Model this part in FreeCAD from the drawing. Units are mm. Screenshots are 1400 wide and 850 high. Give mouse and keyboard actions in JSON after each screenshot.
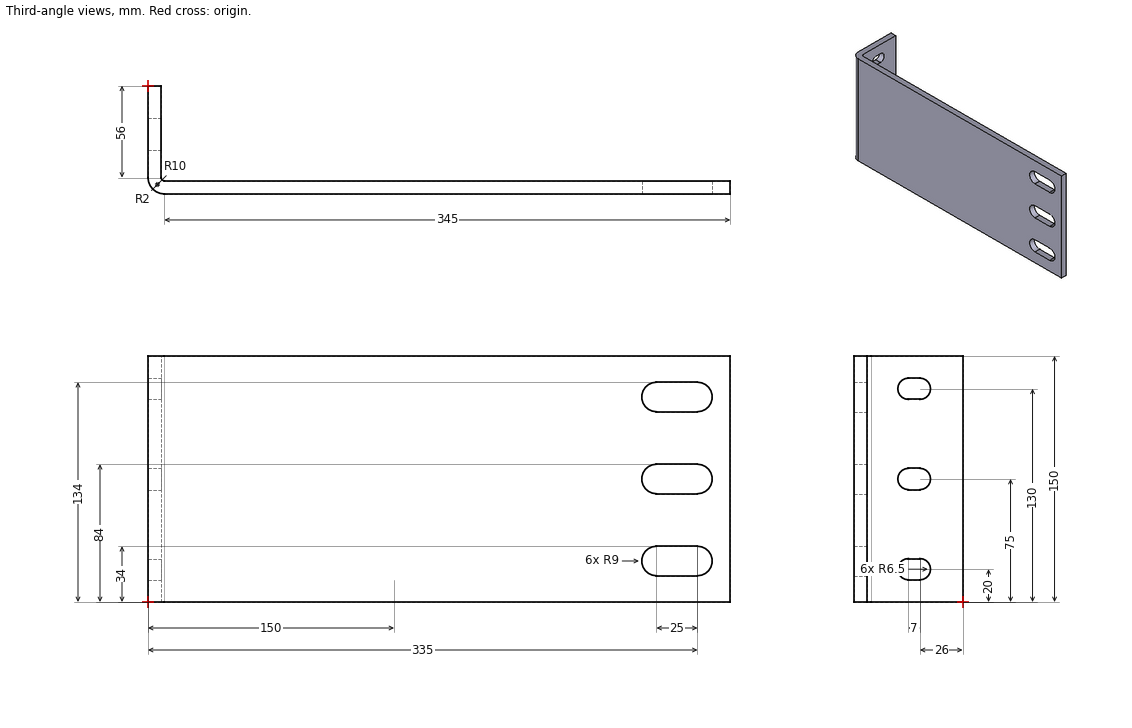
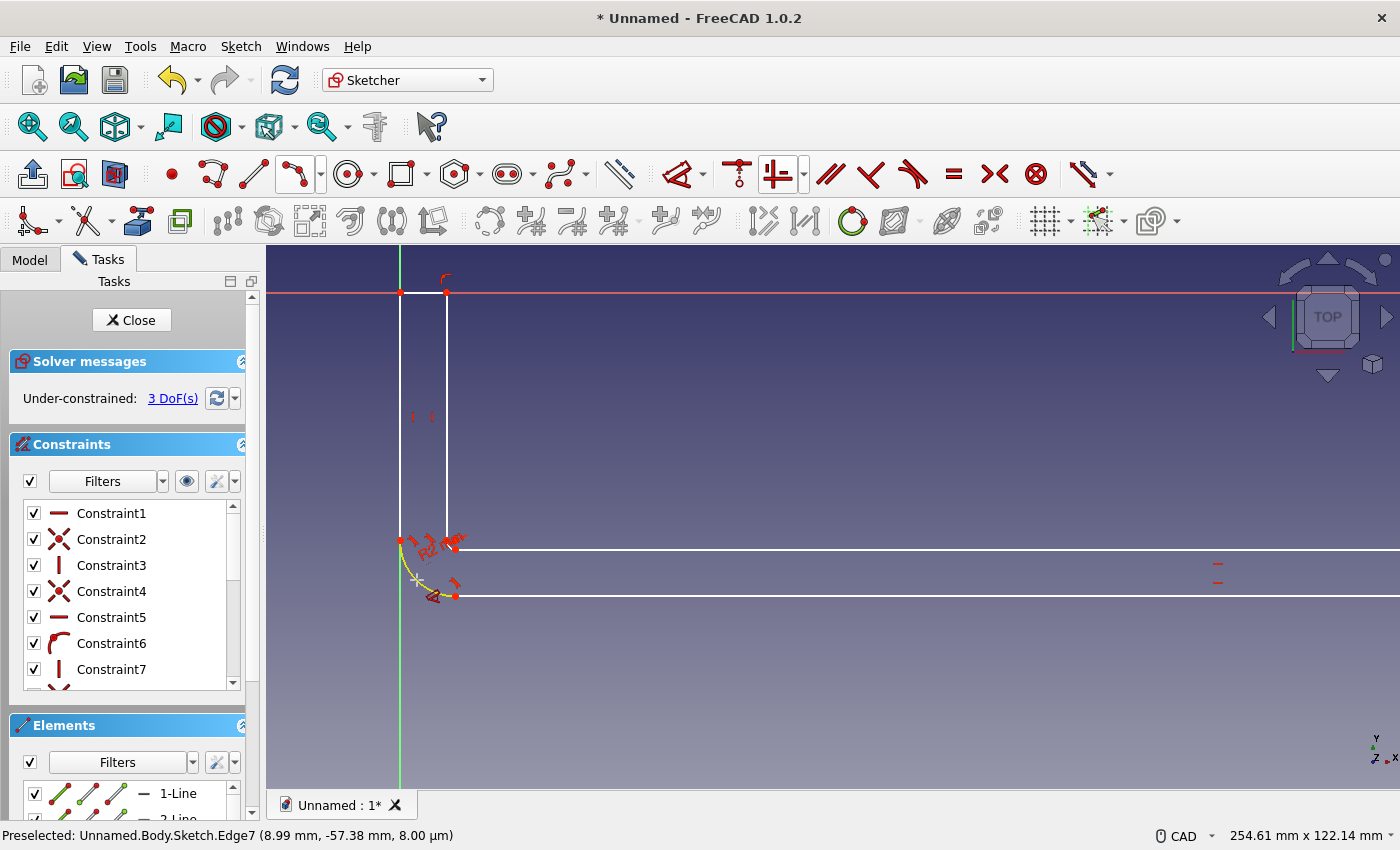
{"action": "left_click", "coordinate": [416, 580]}
{"action": "left_click", "coordinate": [430, 625]}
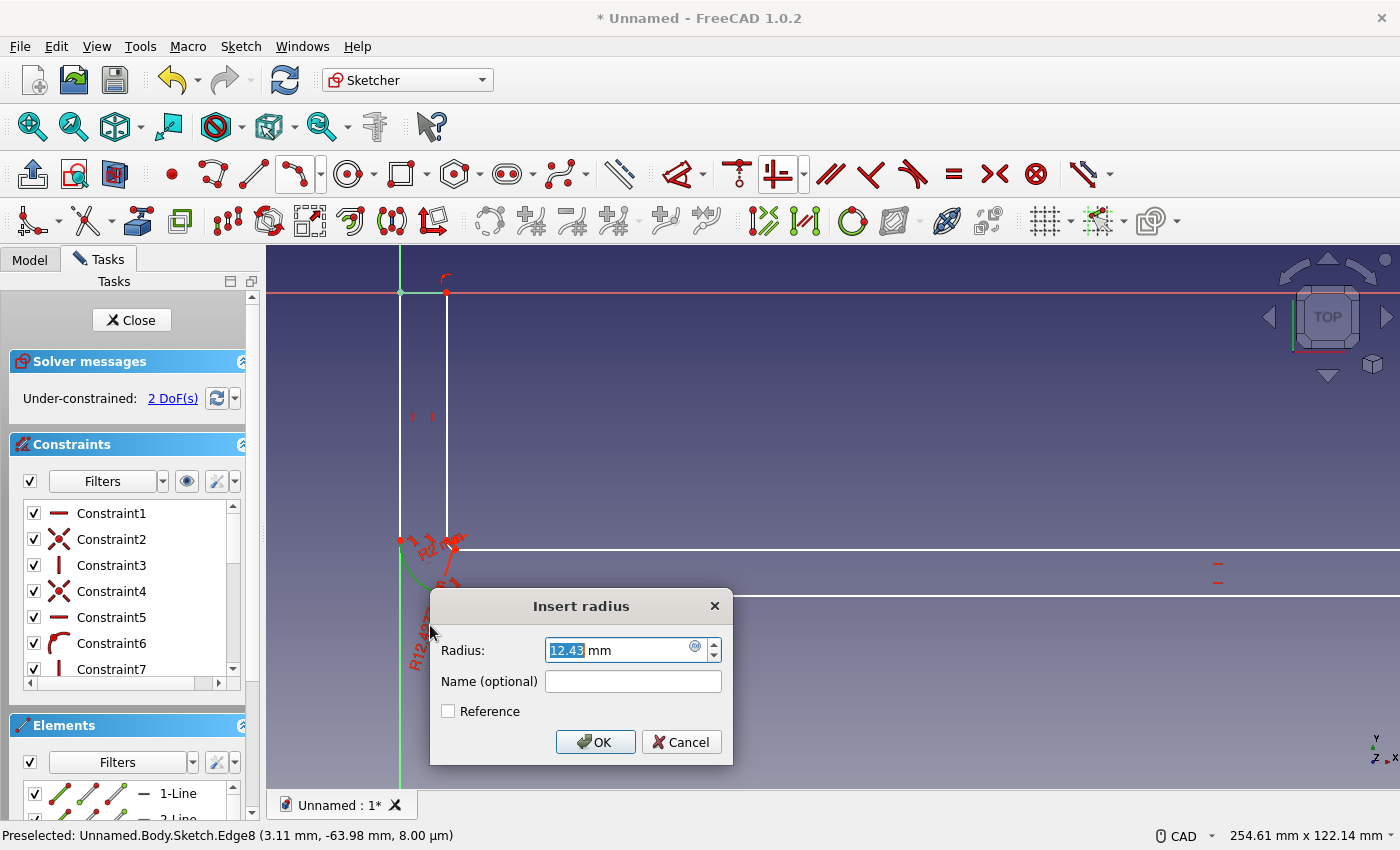
{"action": "type", "text": "10"}
{"action": "key", "text": "Return"}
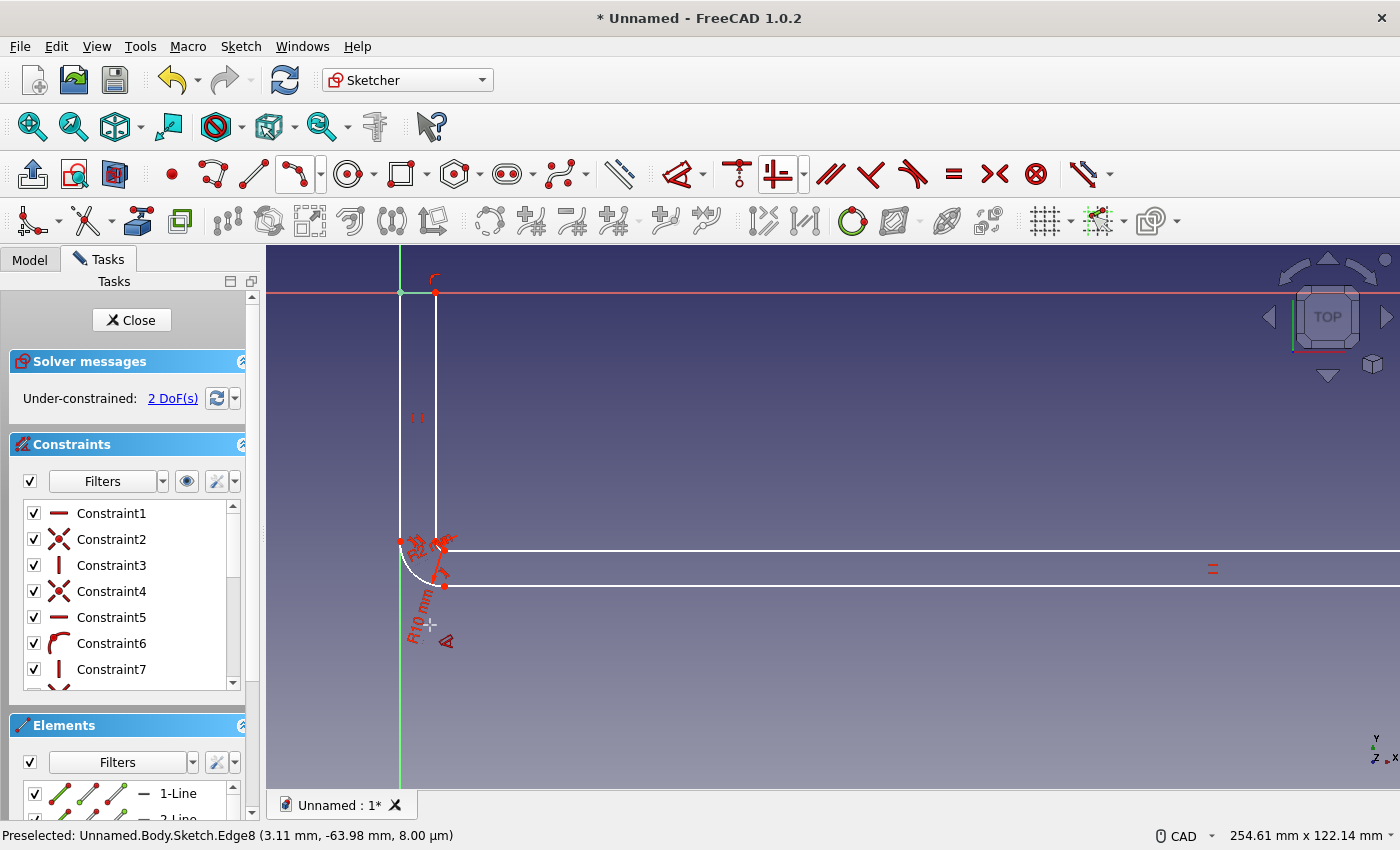
{"action": "left_click", "coordinate": [436, 467]}
{"action": "left_click", "coordinate": [470, 417]}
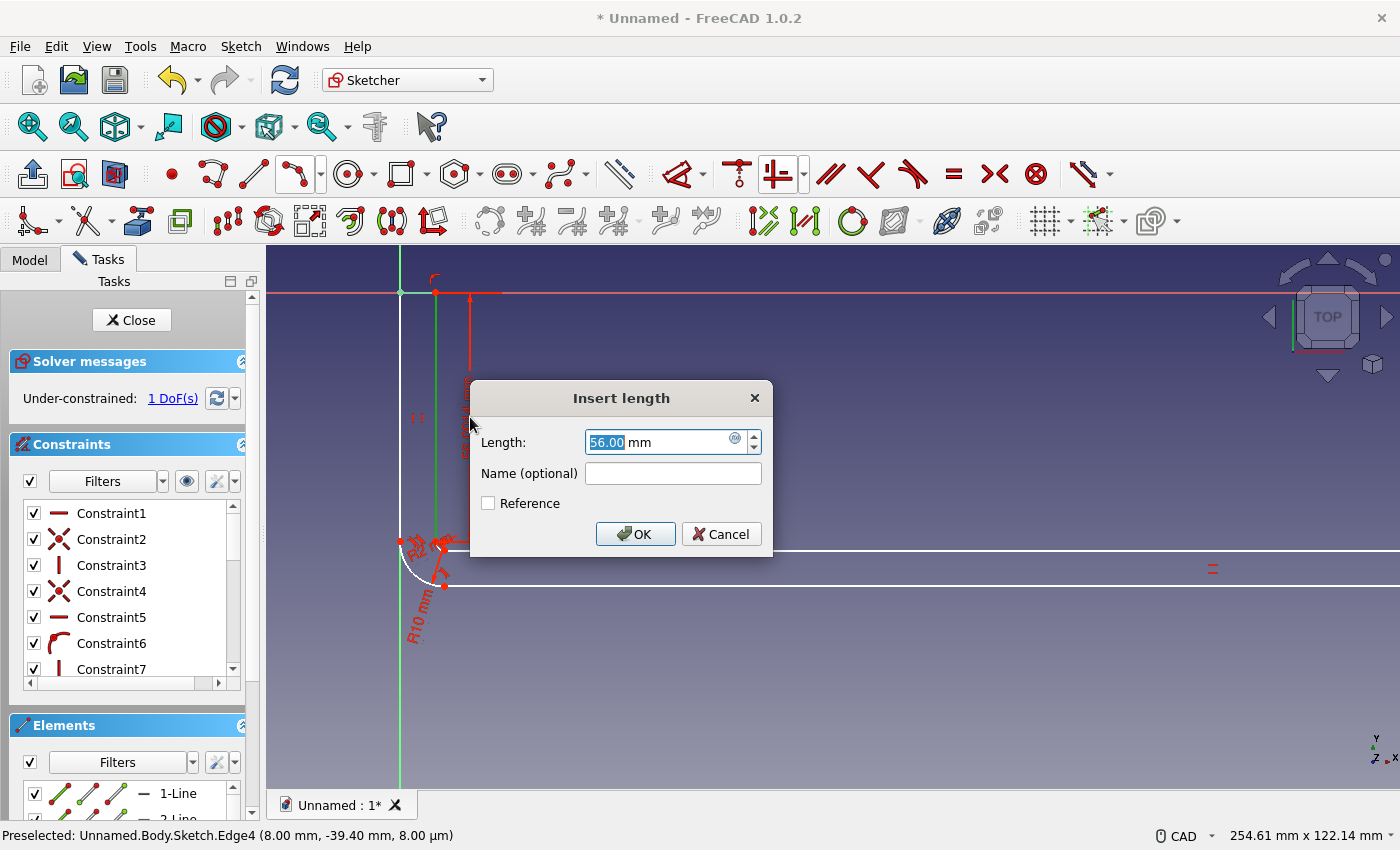
{"action": "type", "text": "56"}
{"action": "key", "text": "Return"}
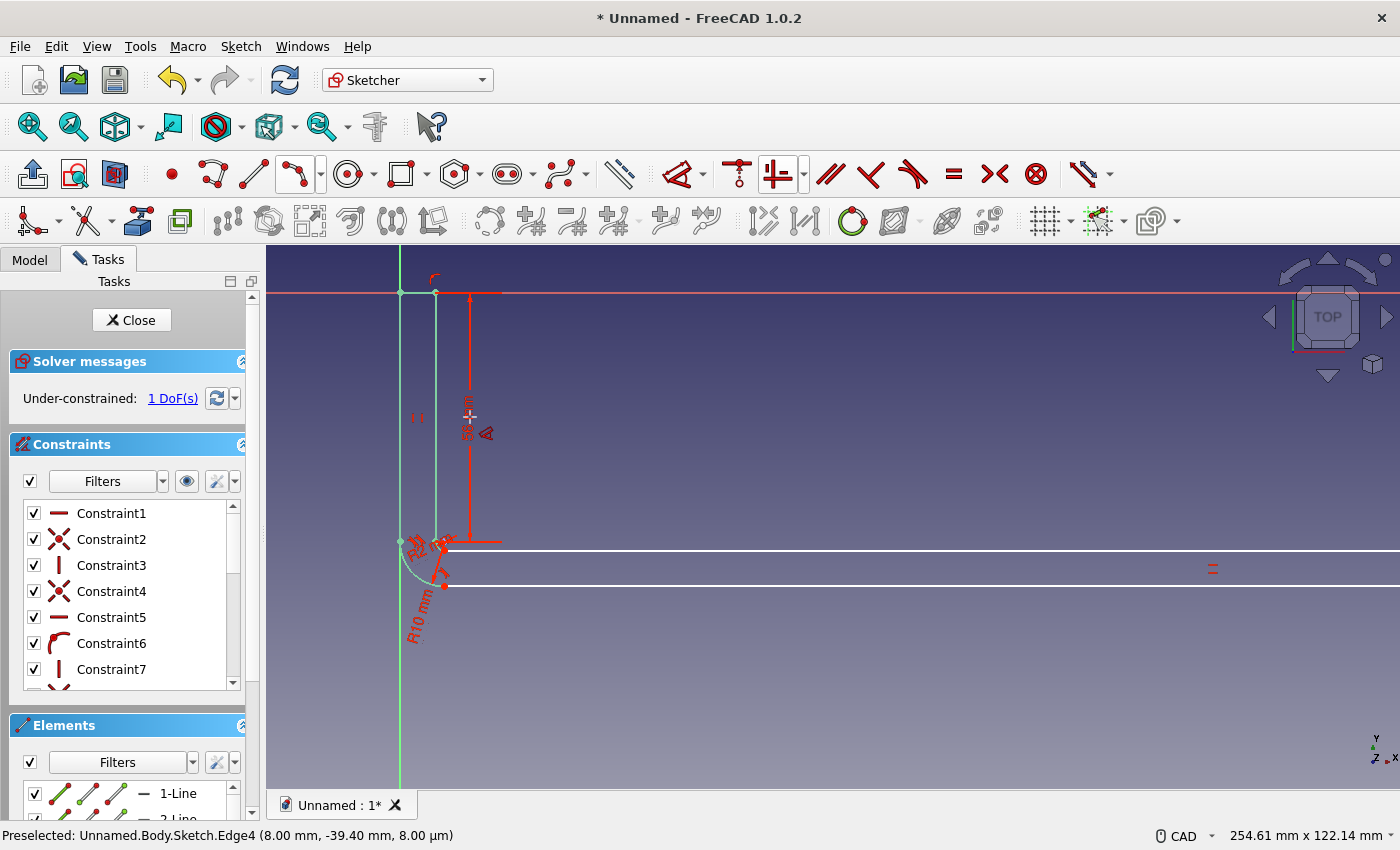
{"action": "left_click", "coordinate": [906, 586]}
{"action": "left_click", "coordinate": [840, 620]}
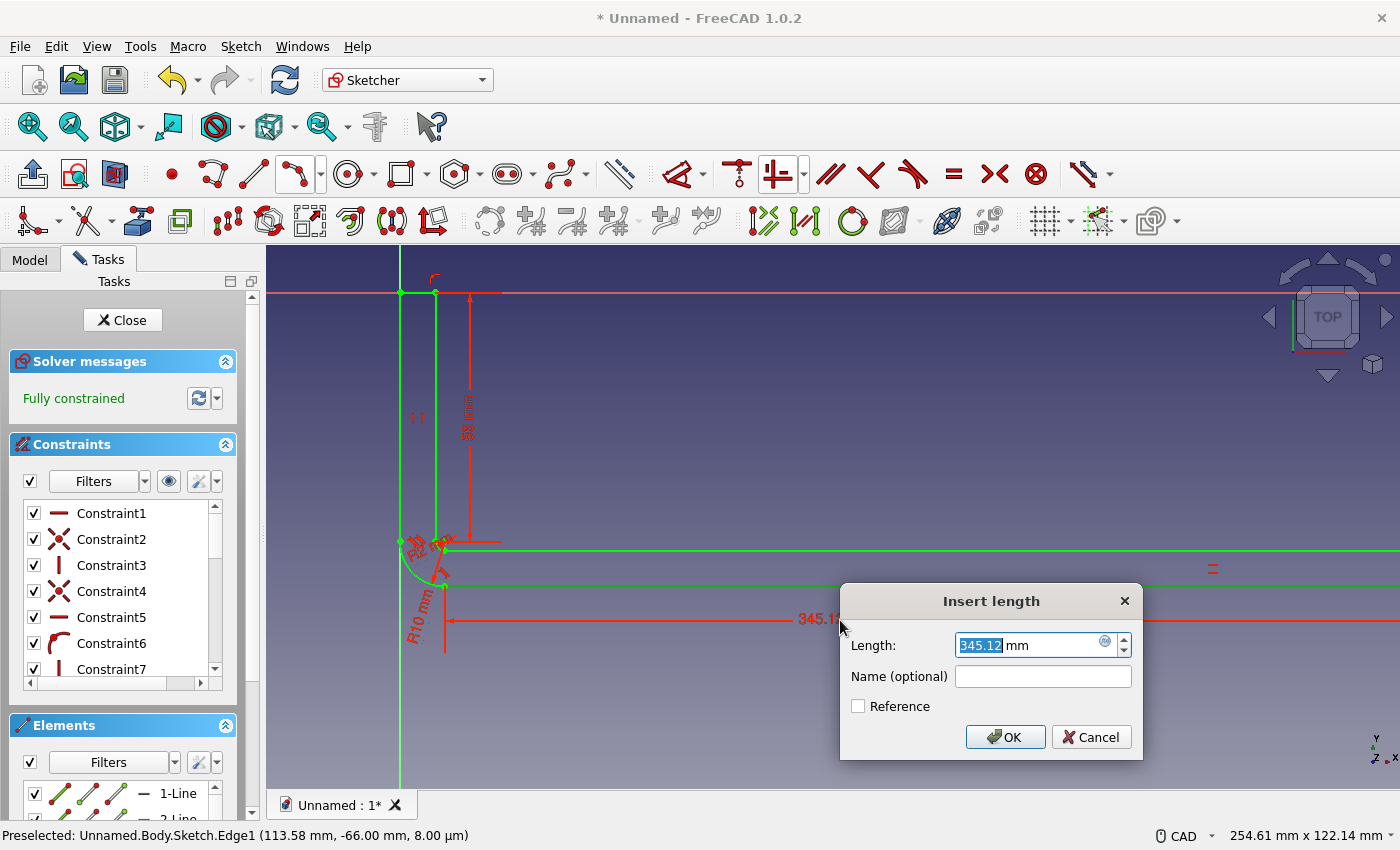
{"action": "type", "text": "345"}
{"action": "key", "text": "Return"}
{"action": "key", "text": "Escape"}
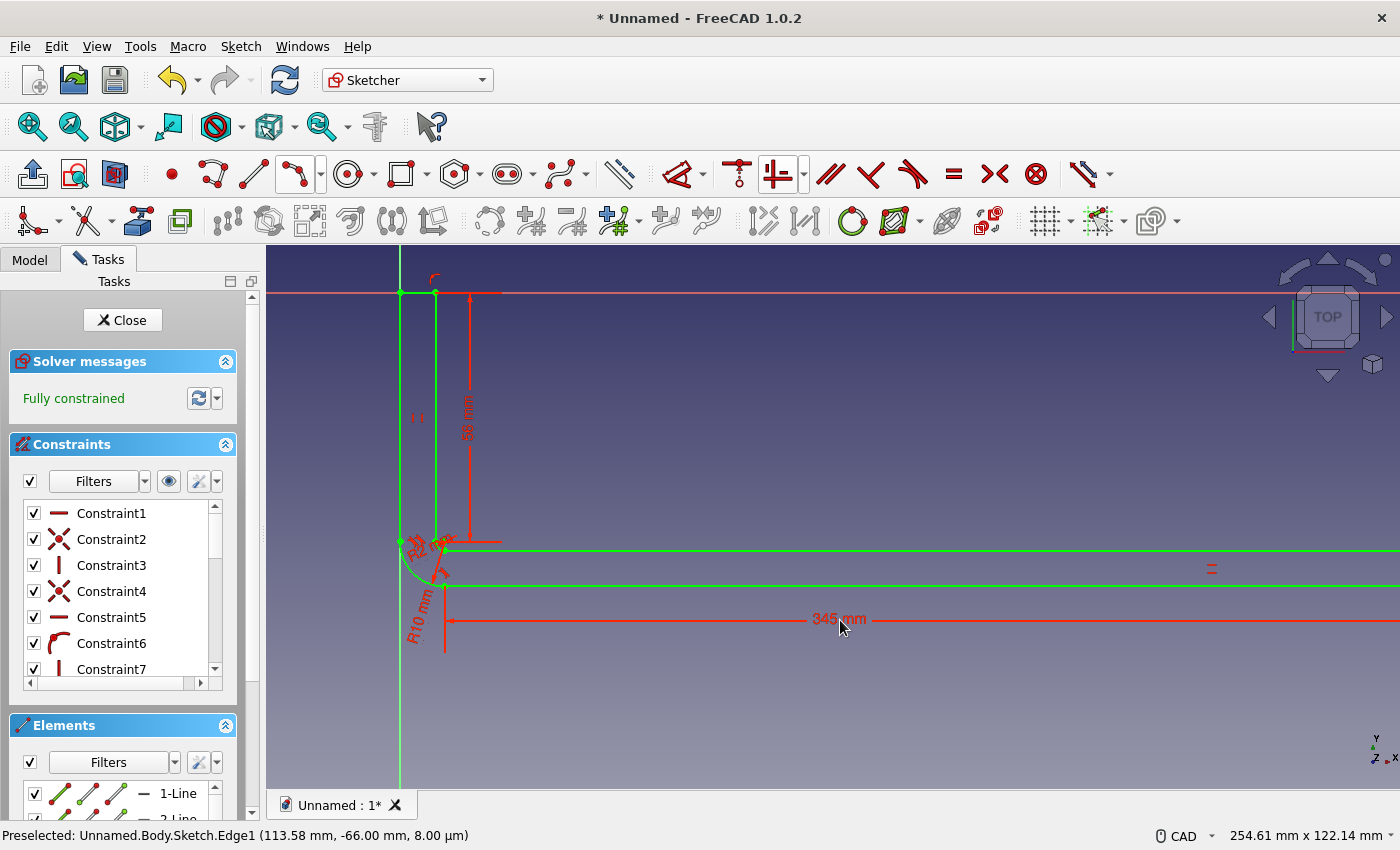
{"action": "left_click", "coordinate": [123, 320]}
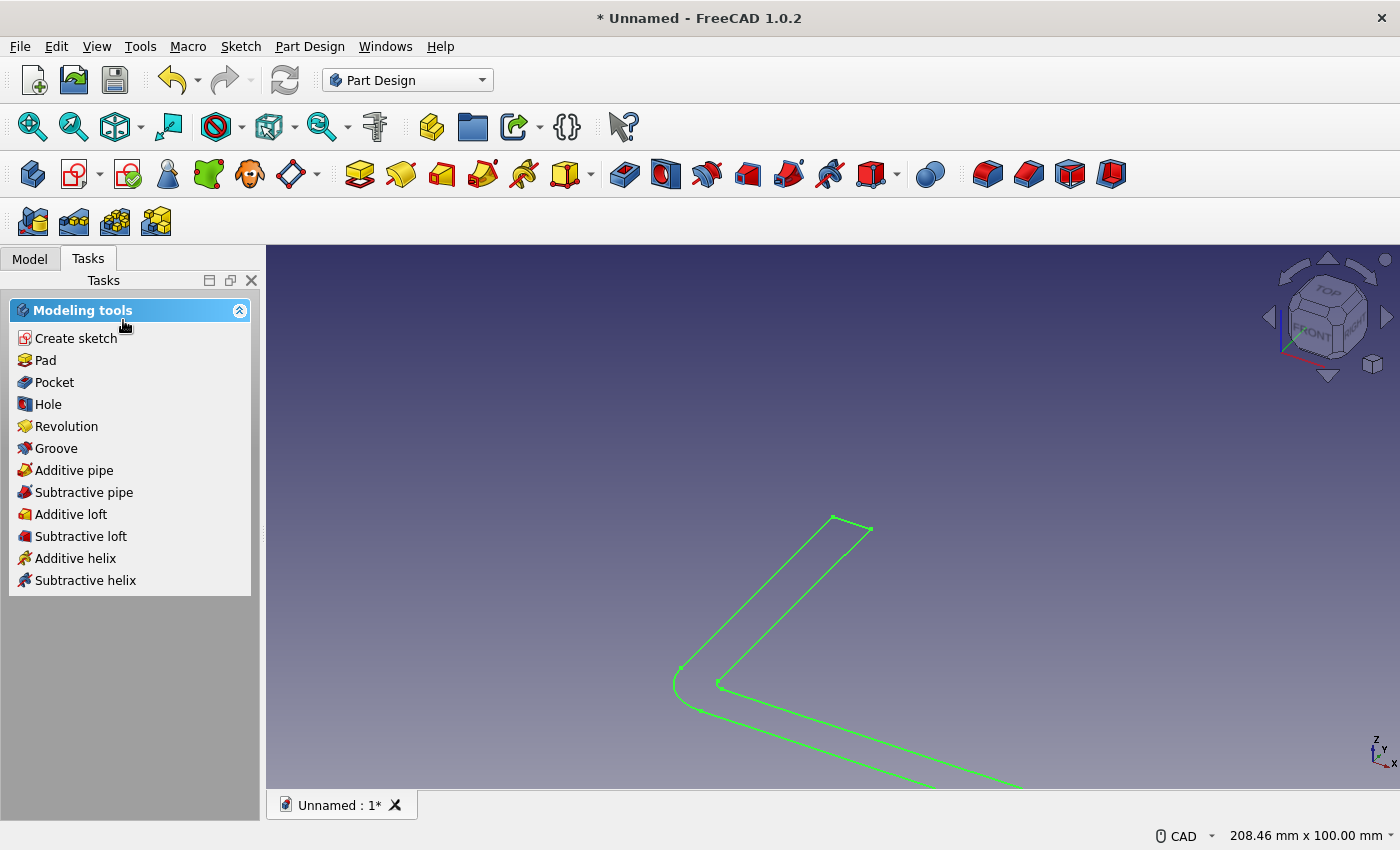
{"action": "left_click", "coordinate": [360, 174]}